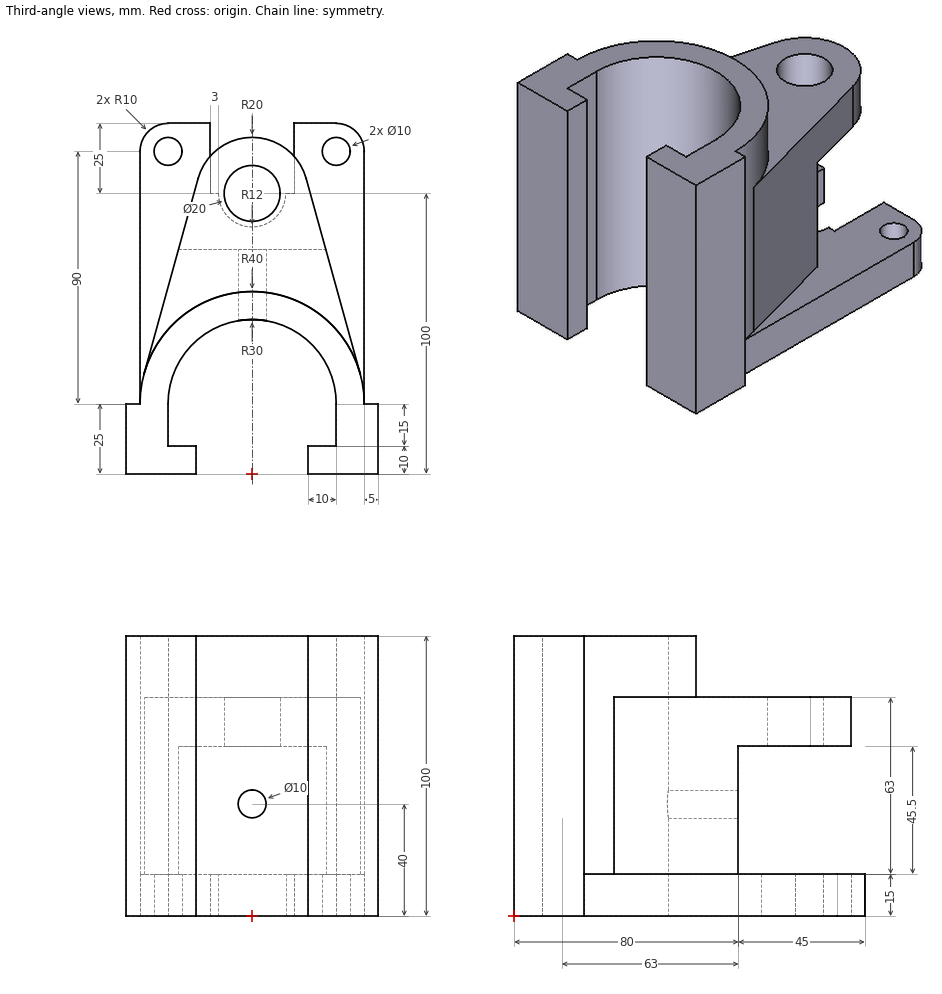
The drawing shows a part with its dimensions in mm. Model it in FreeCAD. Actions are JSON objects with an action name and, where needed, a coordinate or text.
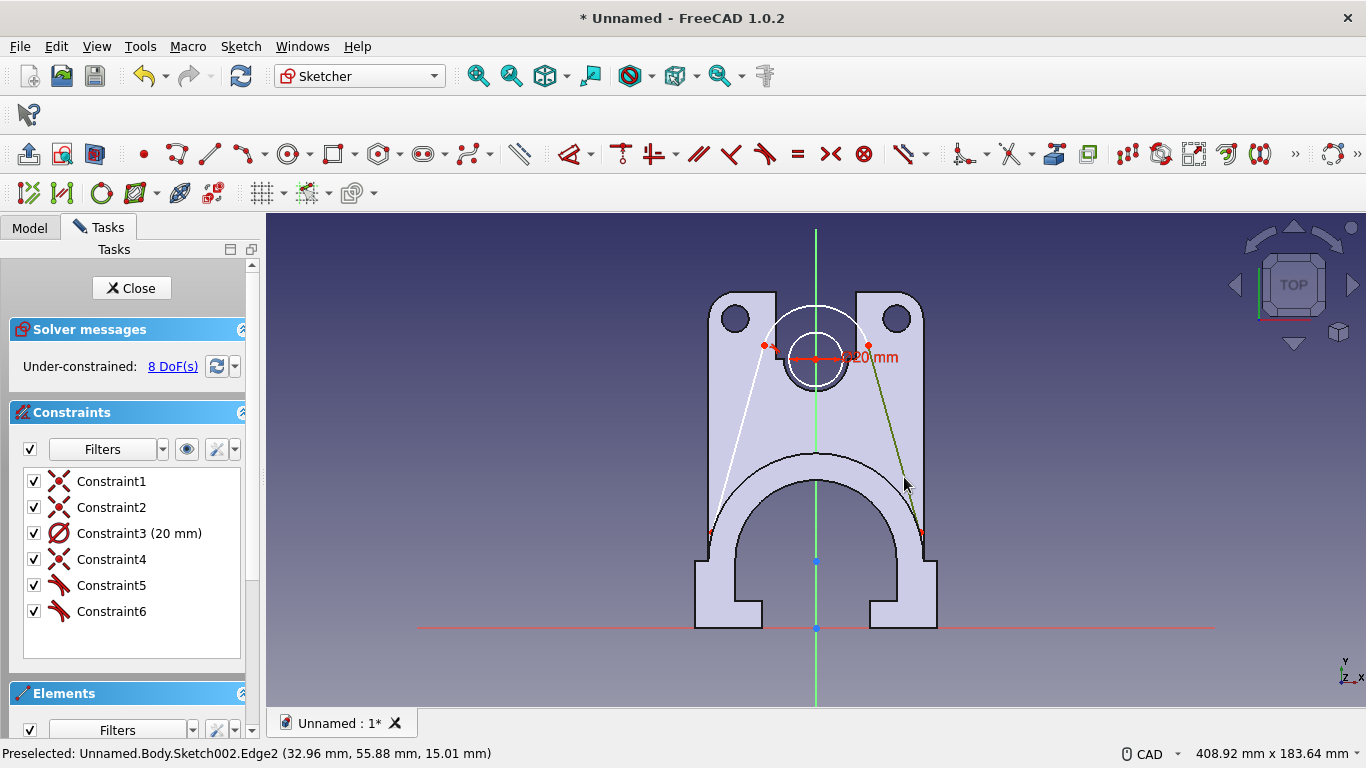
{"action": "left_click", "coordinate": [870, 468]}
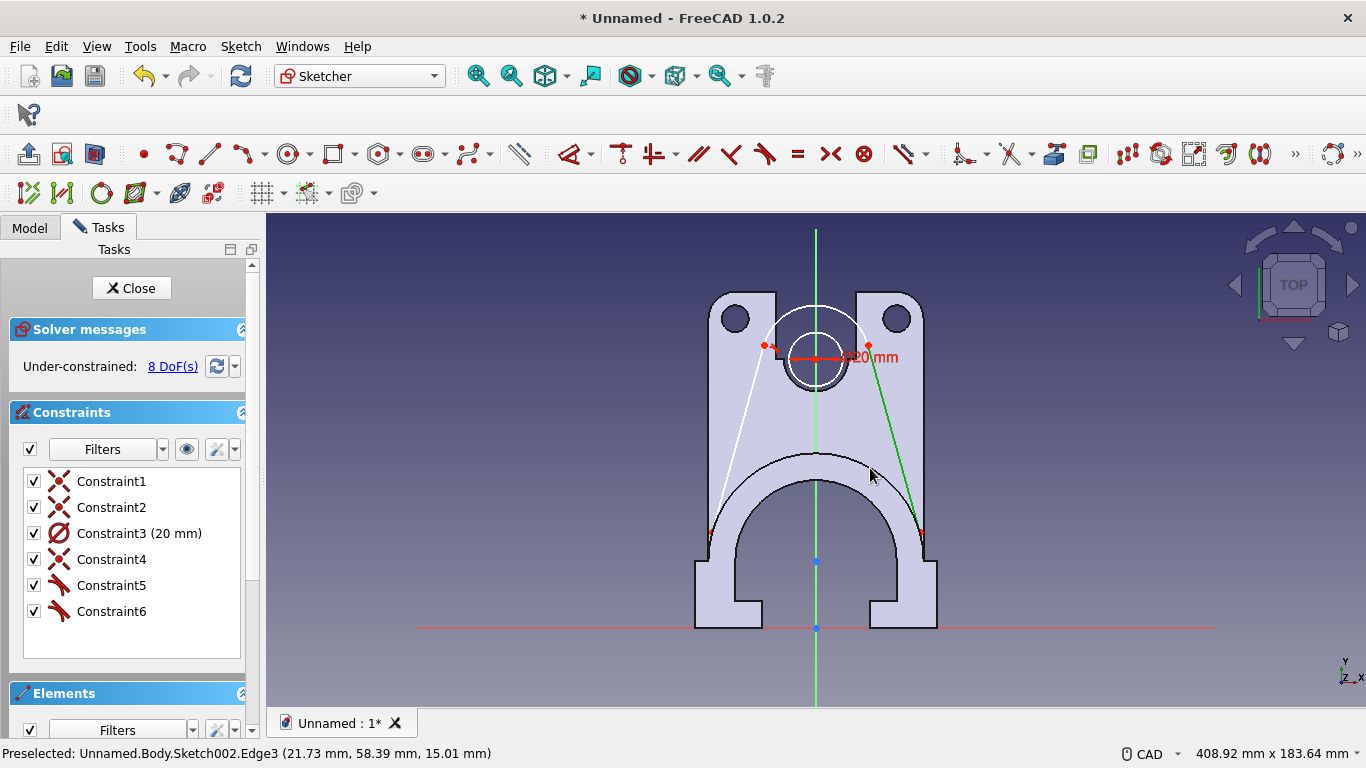
{"action": "key", "text": "t"}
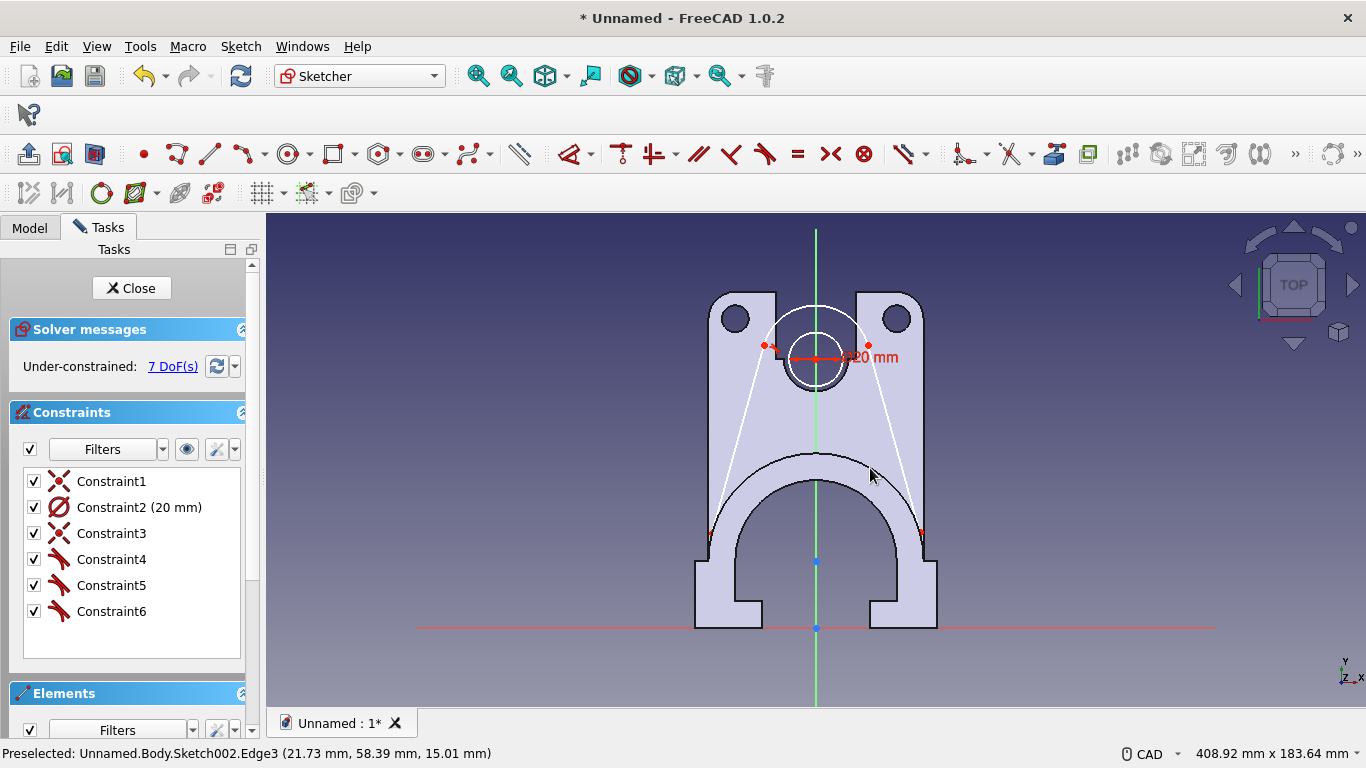
{"action": "left_click", "coordinate": [904, 477]}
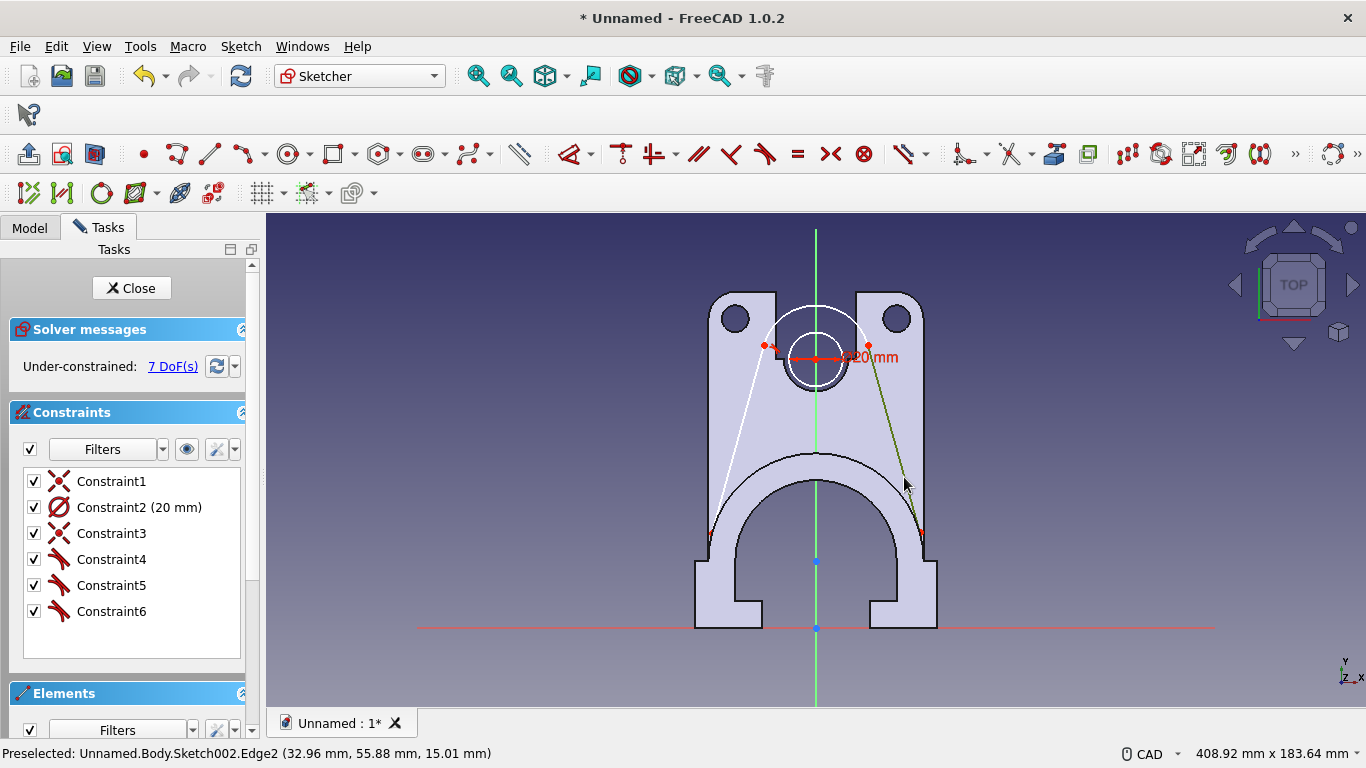
{"action": "left_click", "coordinate": [843, 313]}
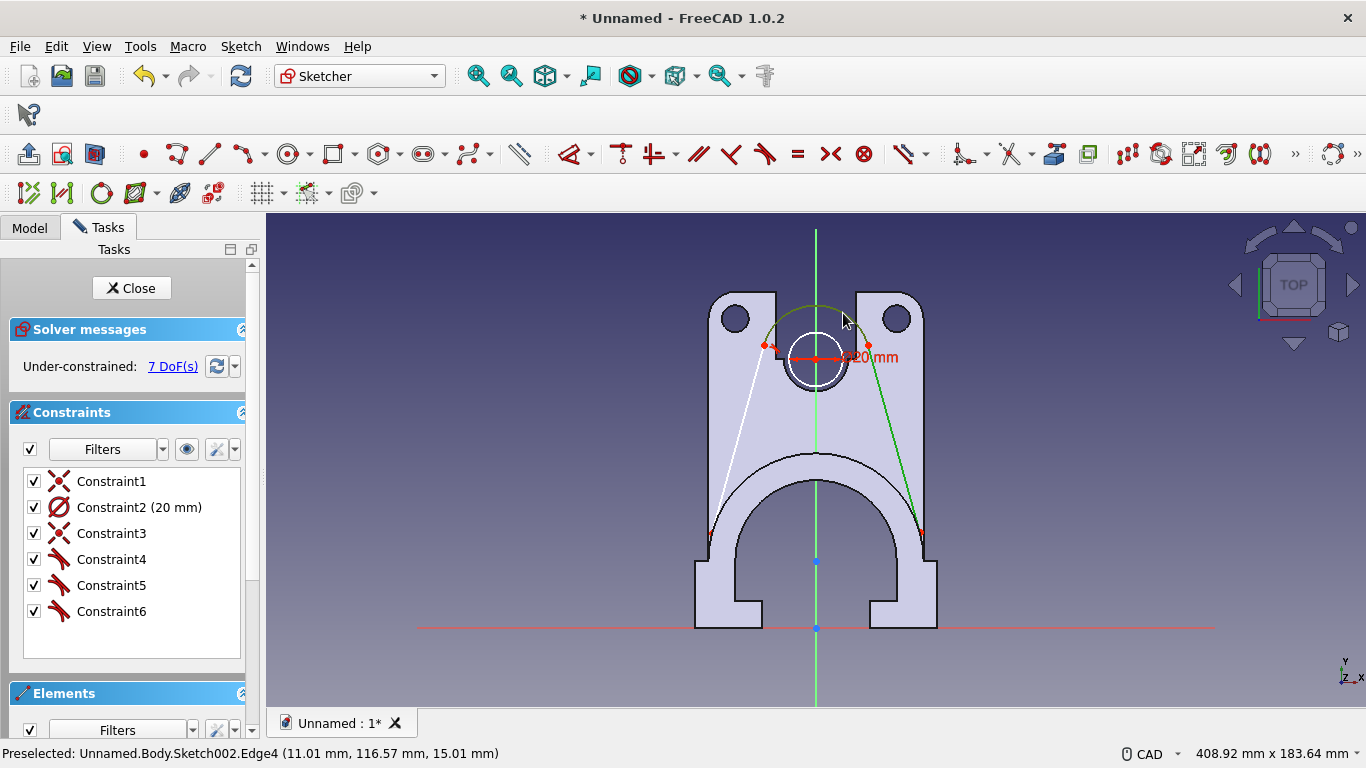
{"action": "key", "text": "t"}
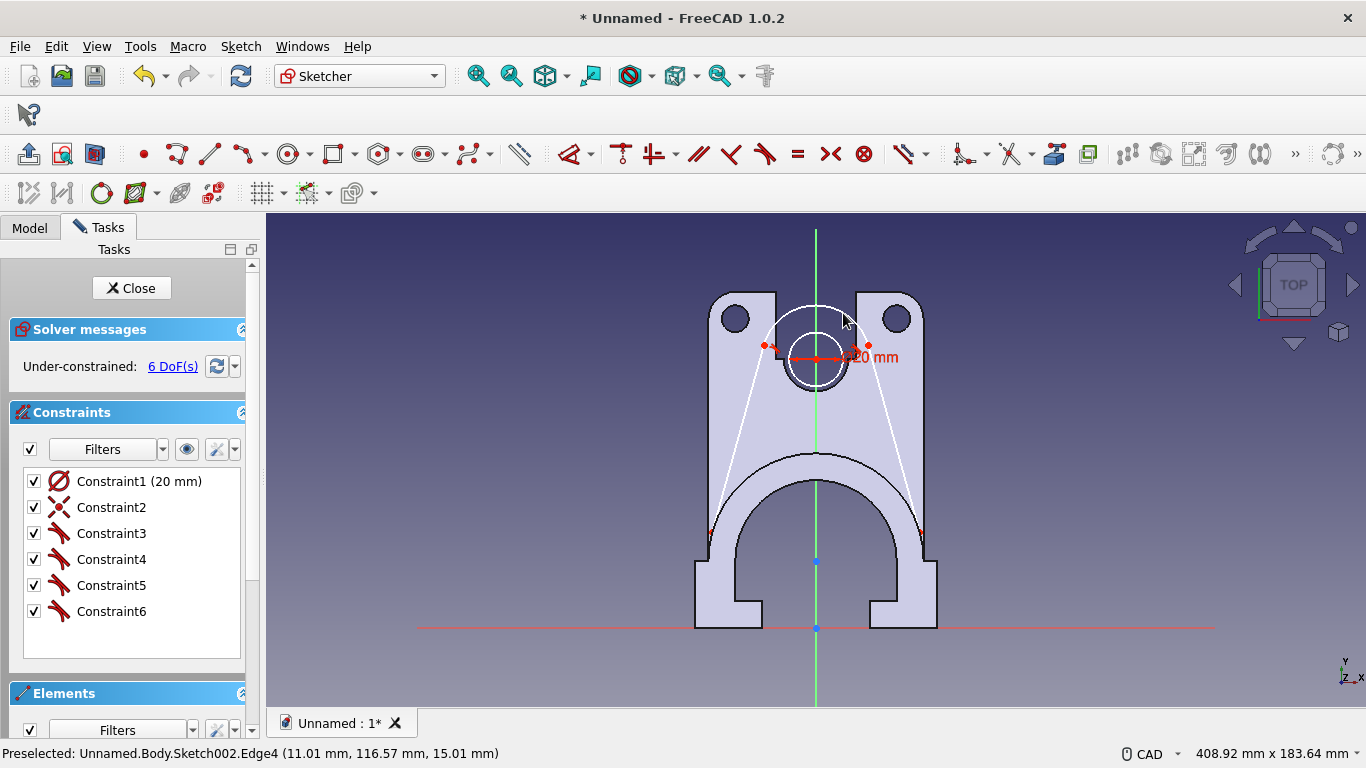
{"action": "left_click", "coordinate": [816, 562]}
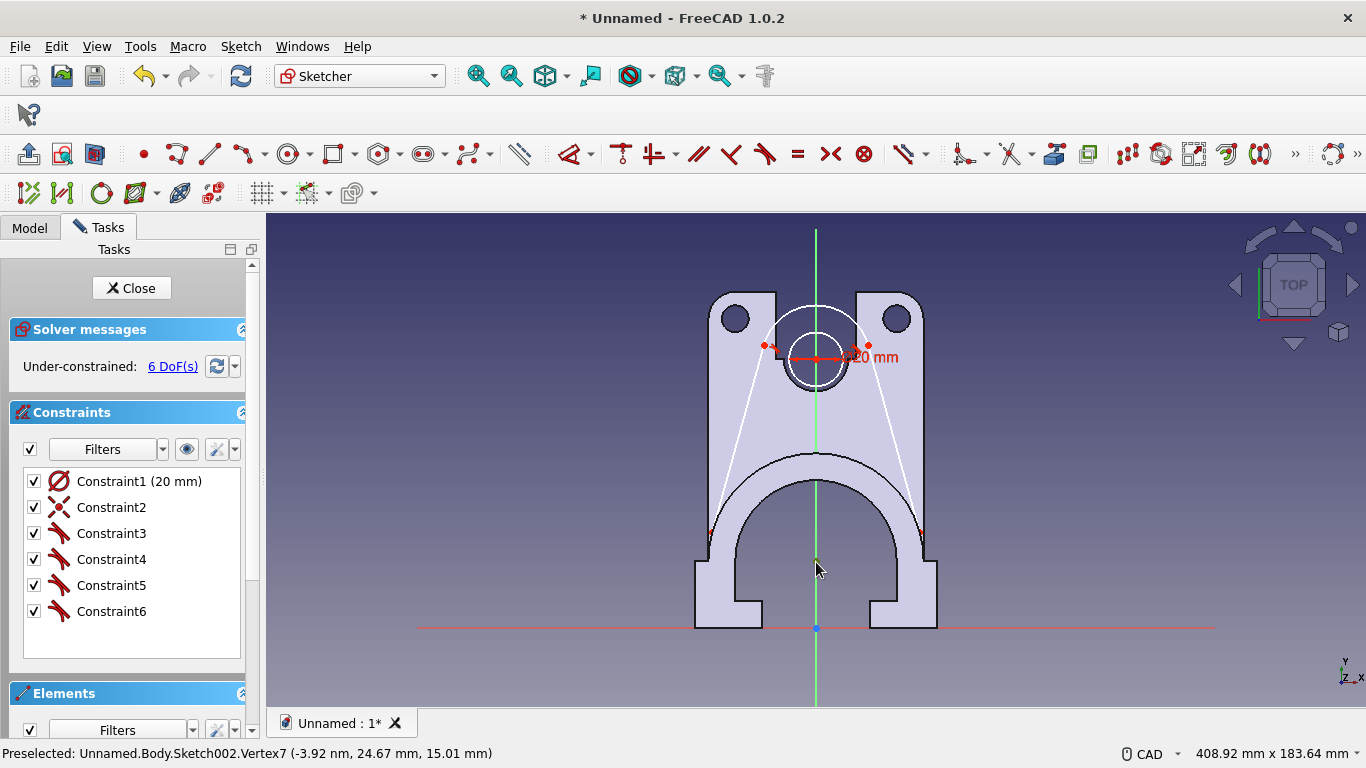
{"action": "left_click", "coordinate": [816, 585]}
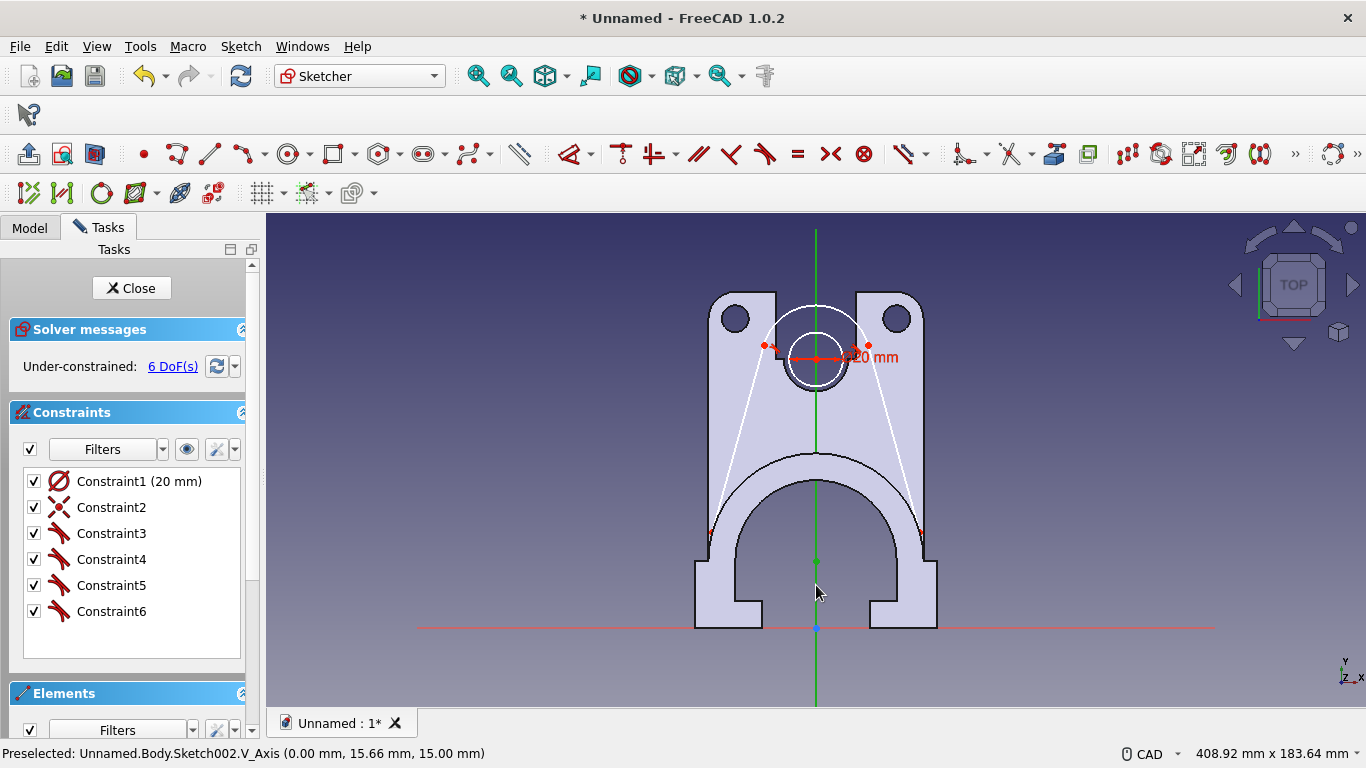
{"action": "key", "text": "c"}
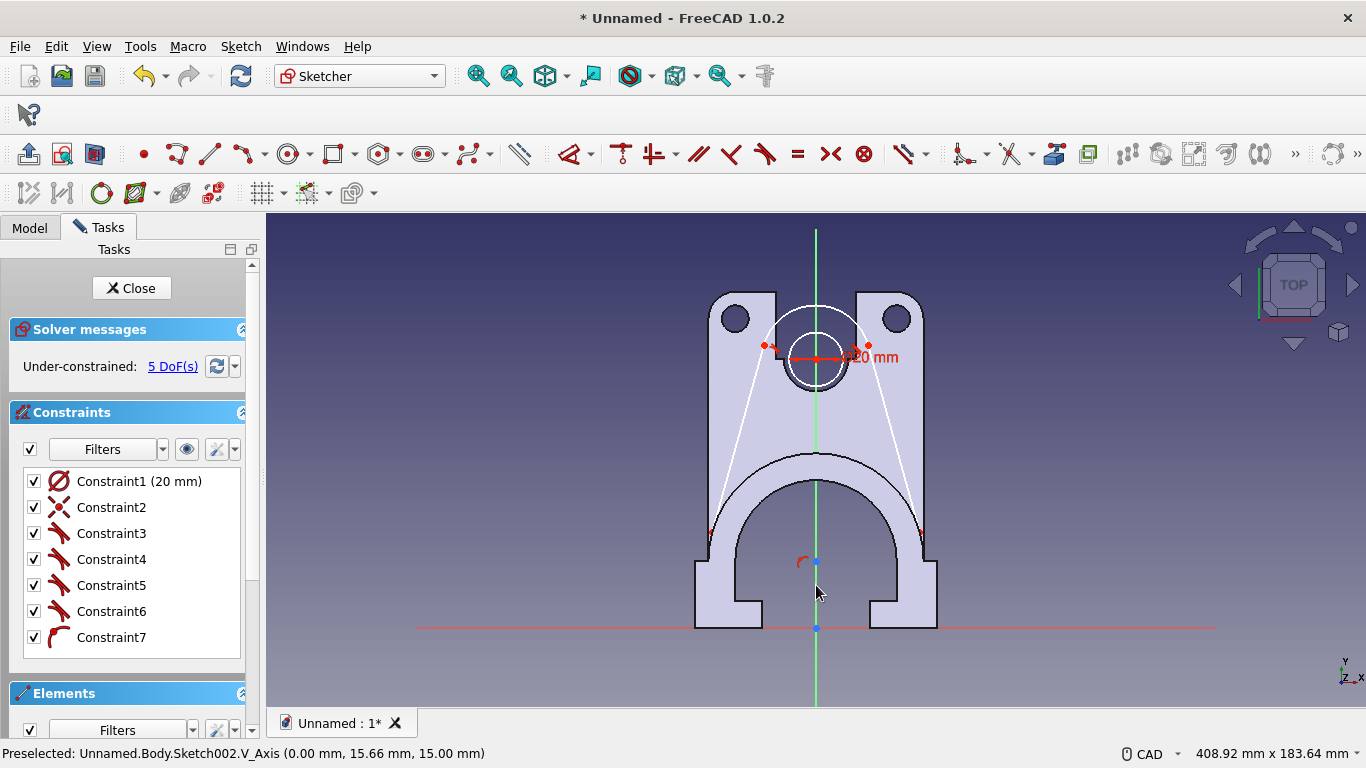
{"action": "left_click", "coordinate": [816, 359]}